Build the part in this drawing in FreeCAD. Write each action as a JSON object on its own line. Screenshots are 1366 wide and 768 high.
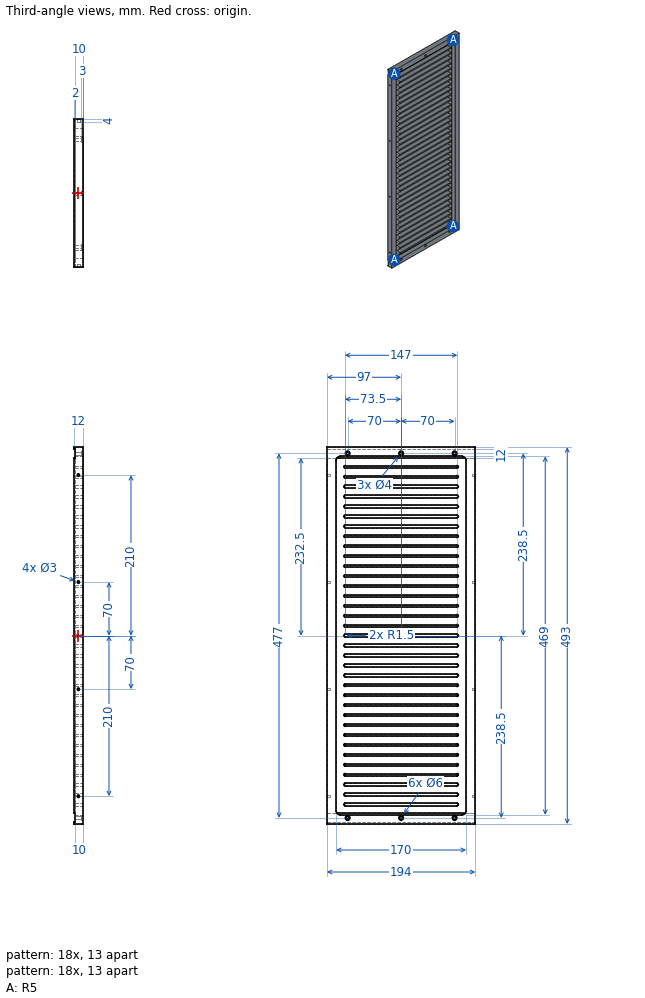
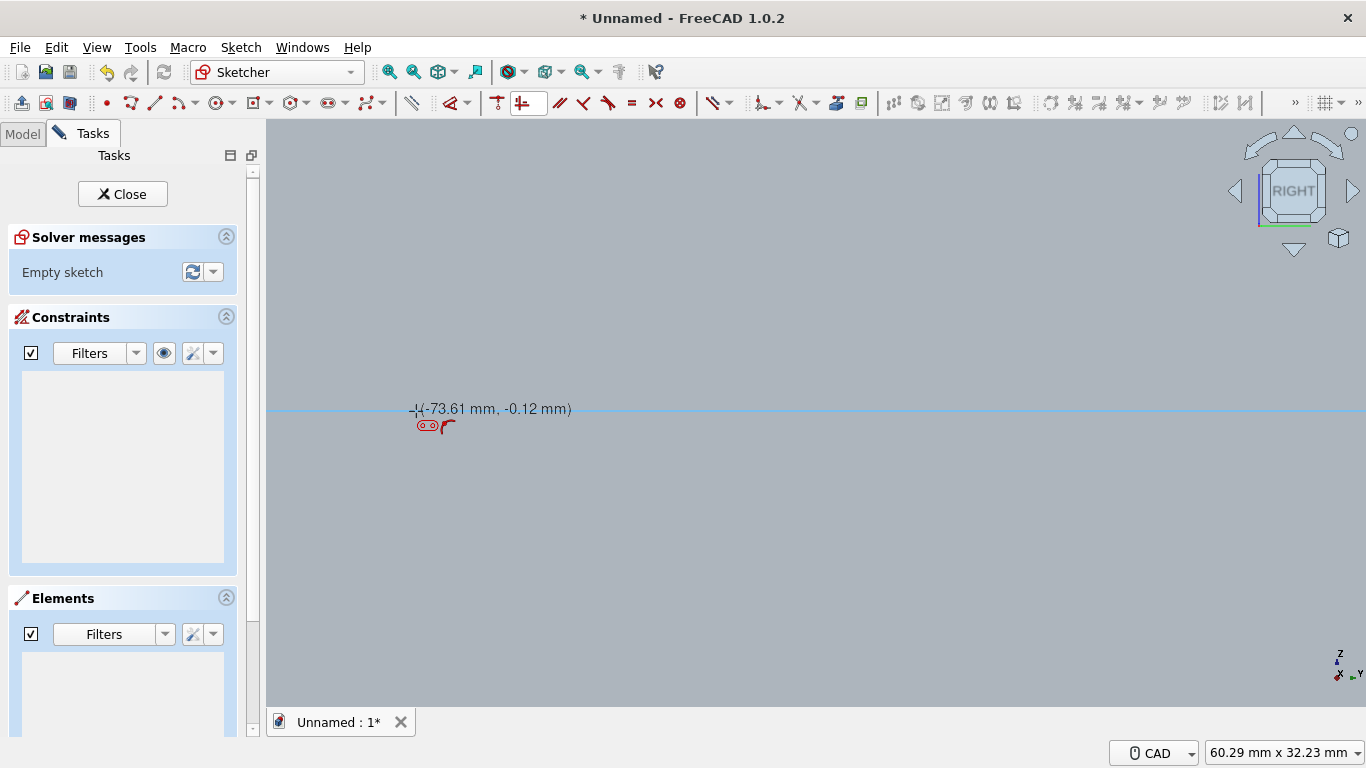
{"action": "scroll", "coordinate": [417, 414], "scroll_direction": "down", "scroll_amount": 7}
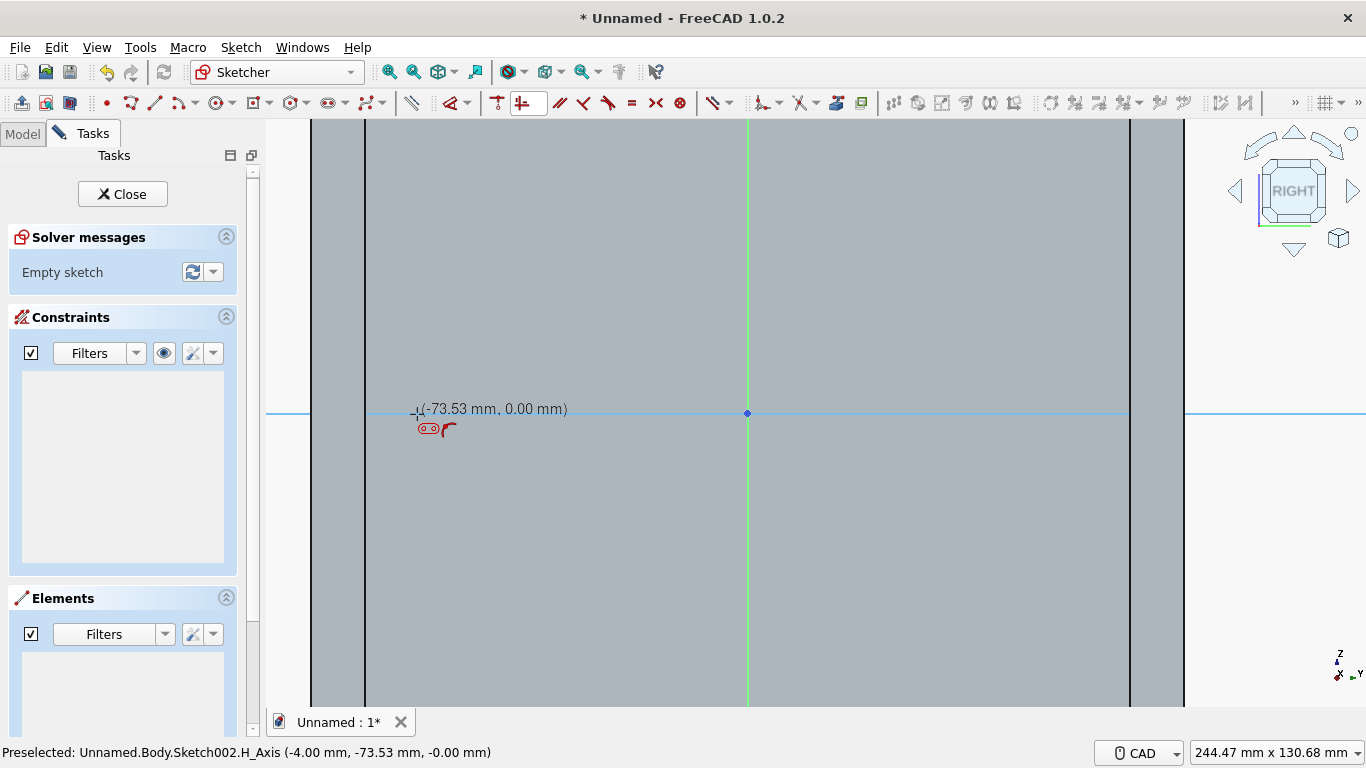
{"action": "left_click", "coordinate": [417, 414]}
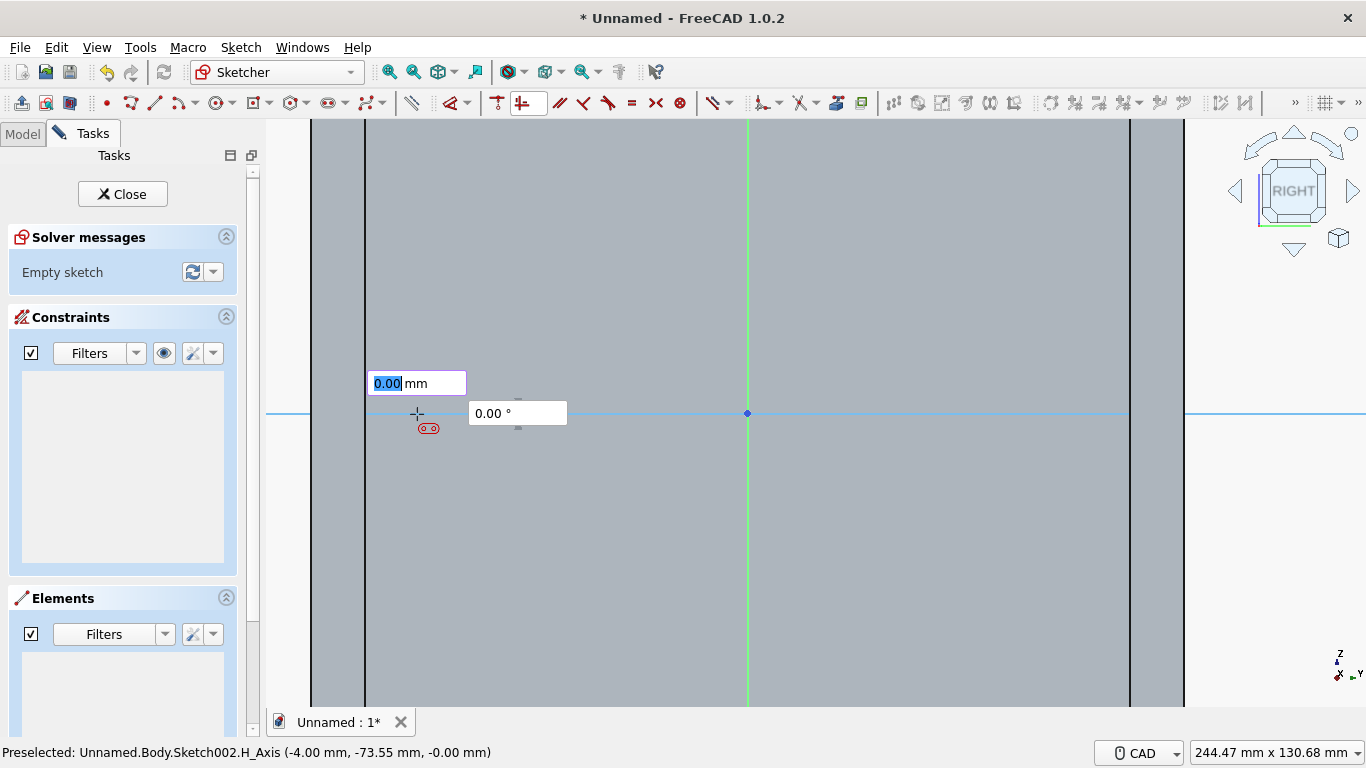
{"action": "left_click", "coordinate": [1079, 405]}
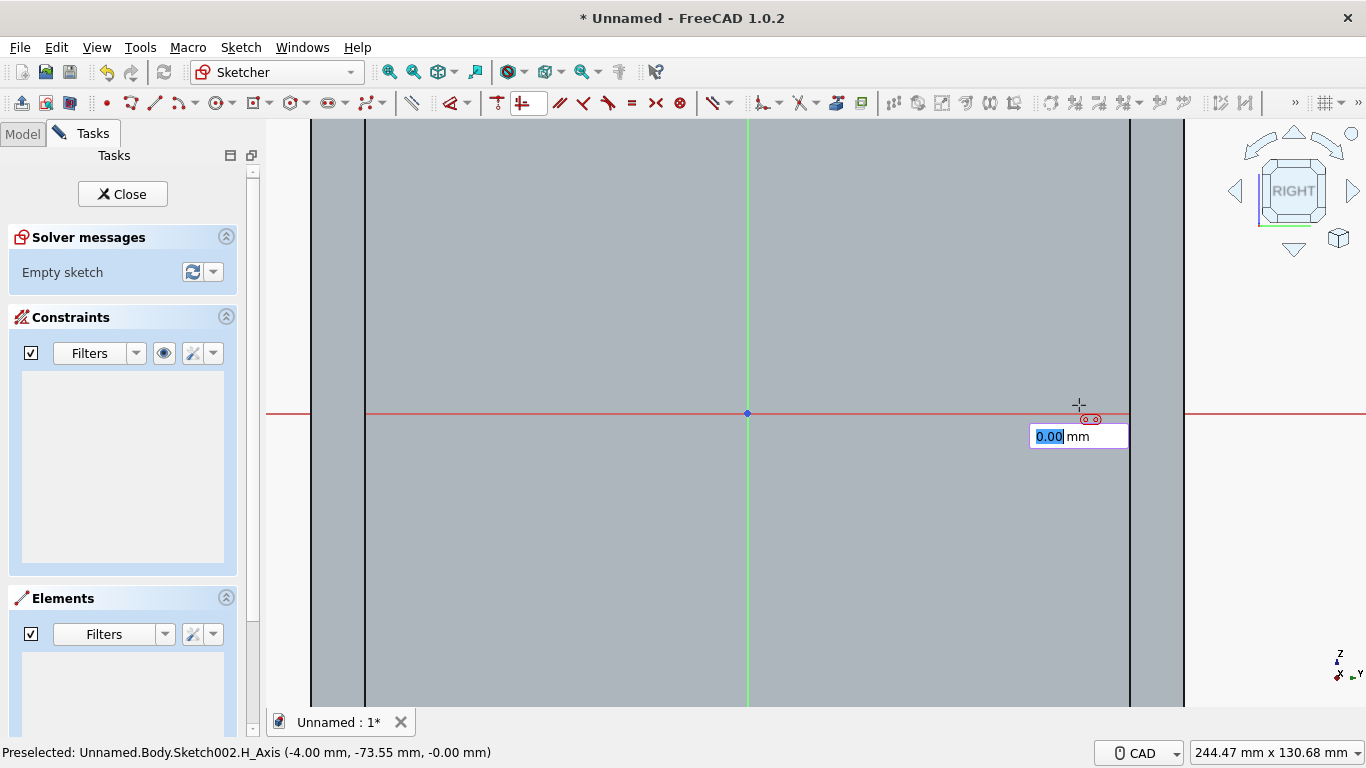
{"action": "scroll", "coordinate": [847, 407], "scroll_direction": "up", "scroll_amount": 5}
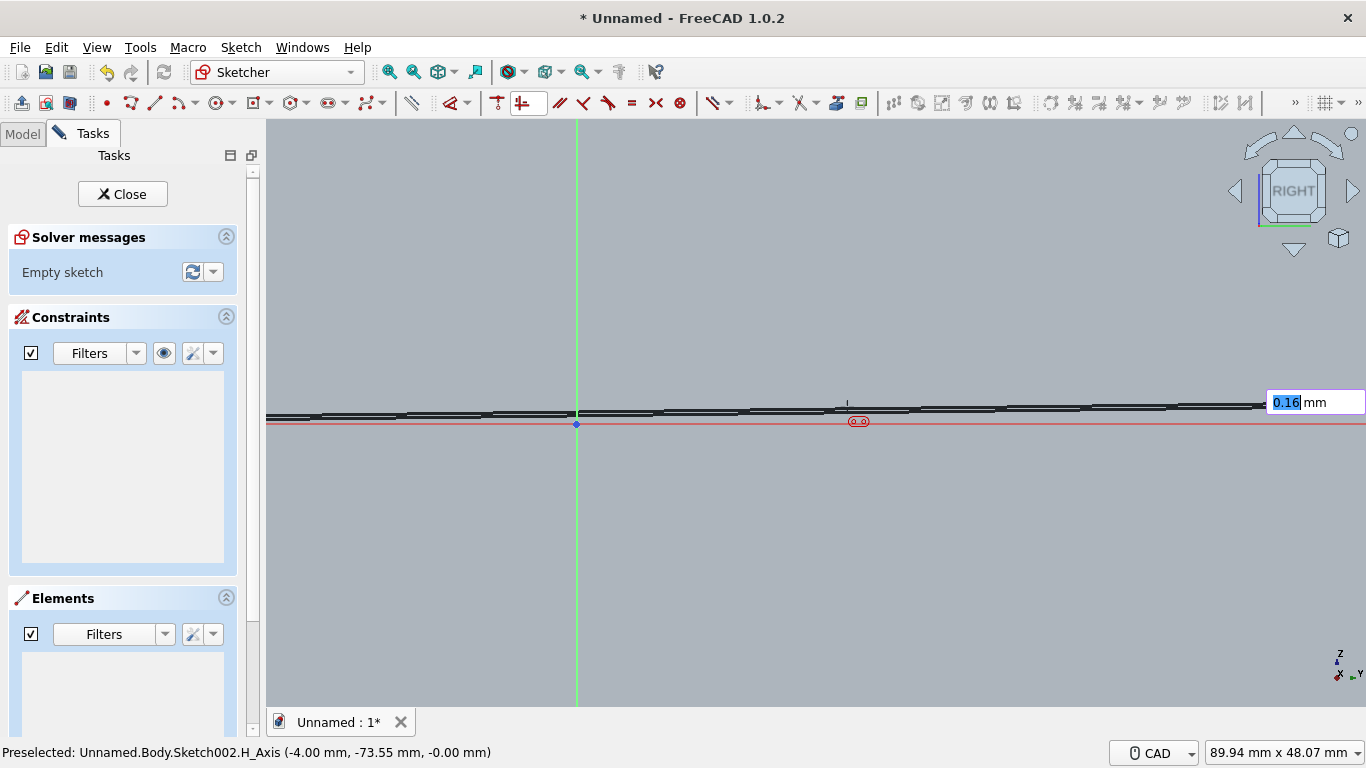
{"action": "left_click", "coordinate": [847, 406]}
{"action": "key", "text": "Escape"}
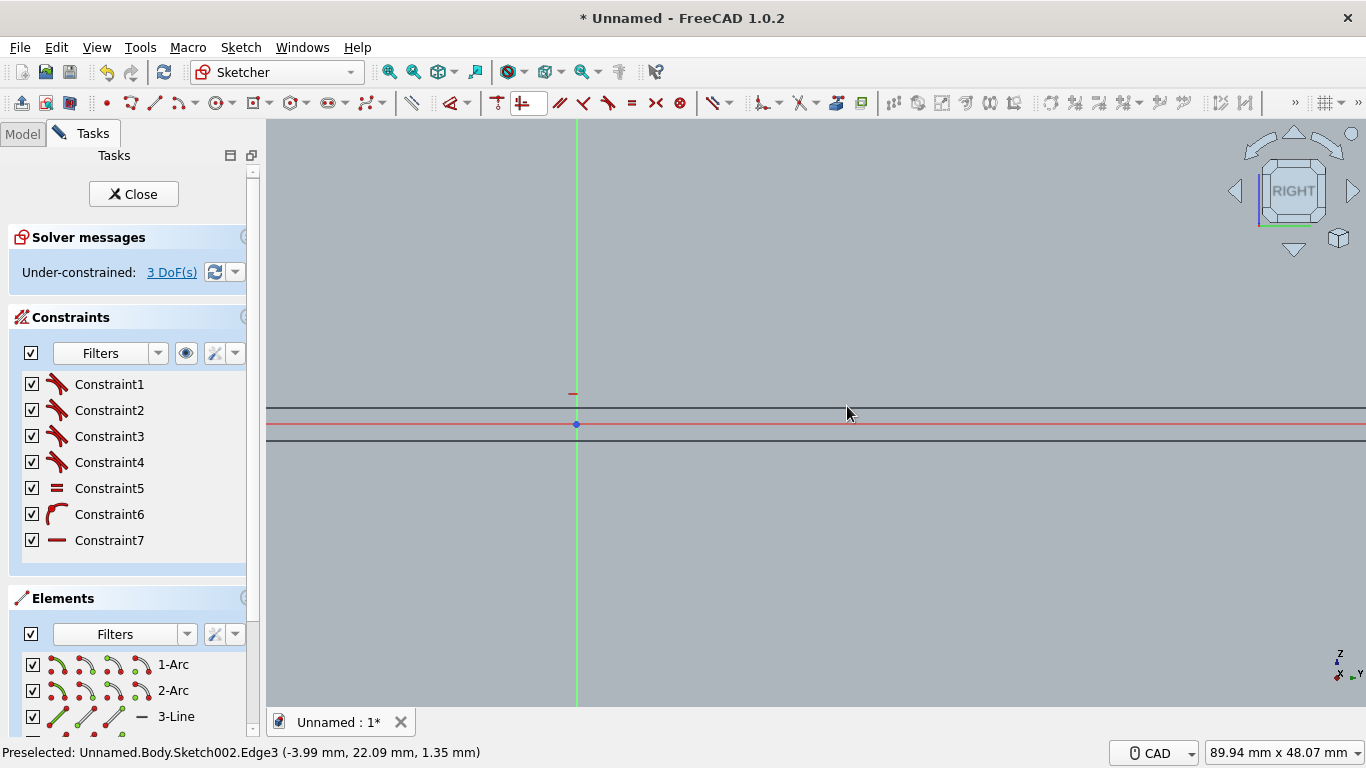
{"action": "scroll", "coordinate": [847, 406], "scroll_direction": "down", "scroll_amount": 5}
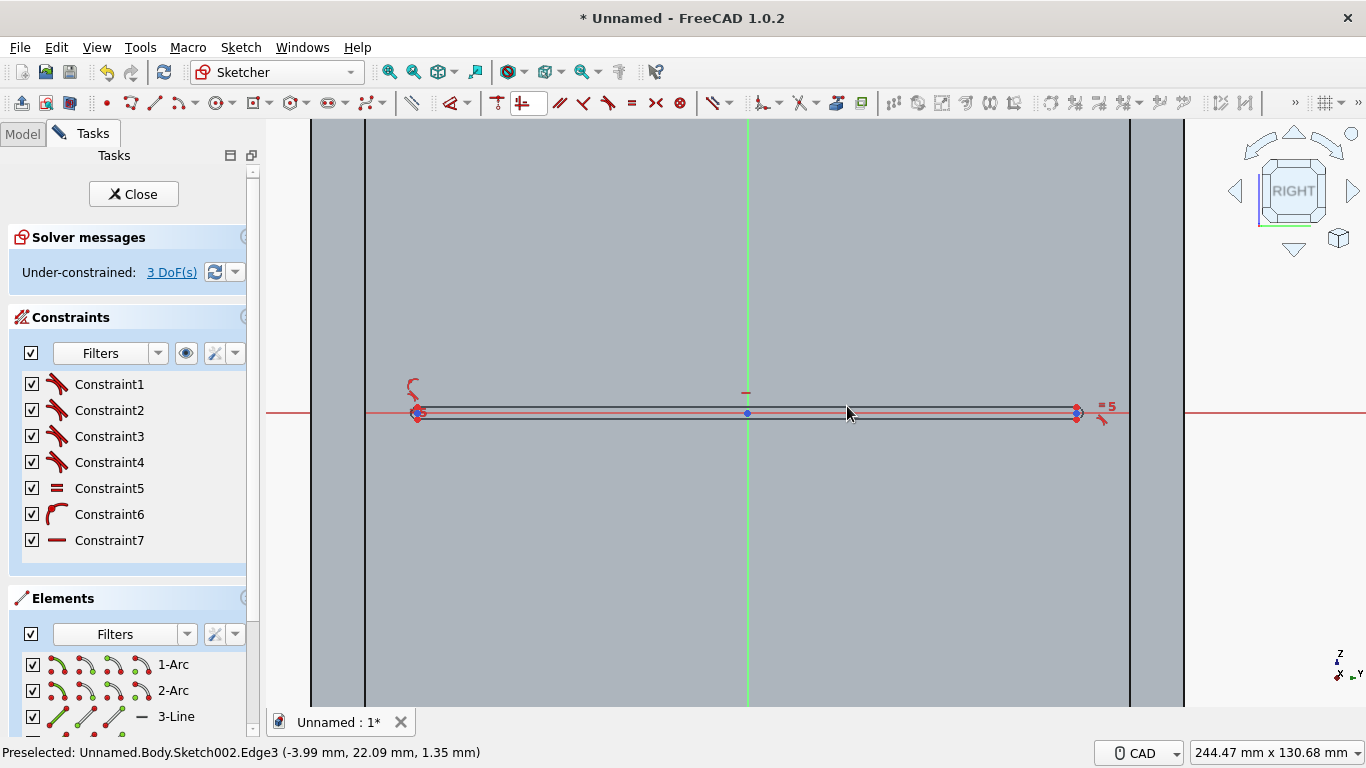
{"action": "scroll", "coordinate": [412, 410], "scroll_direction": "up", "scroll_amount": 9}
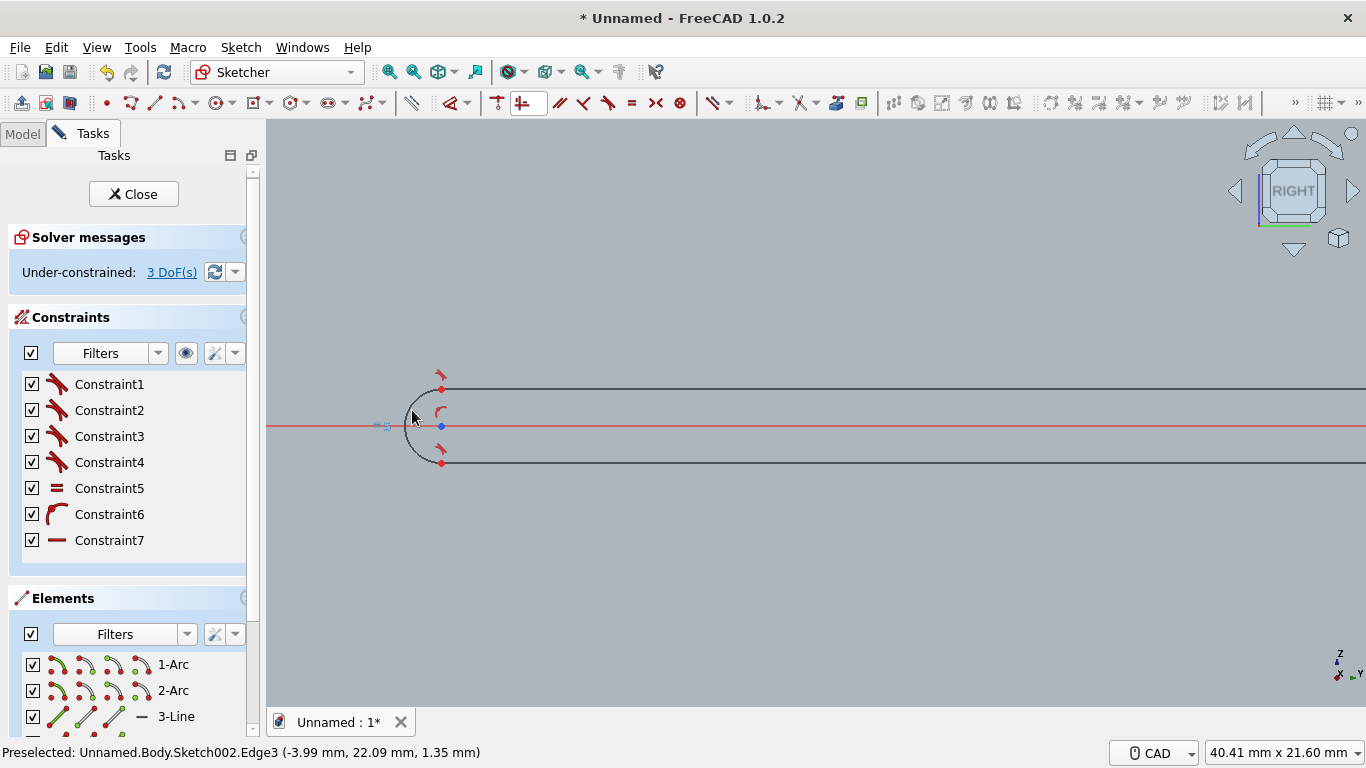
{"action": "left_click", "coordinate": [412, 405]}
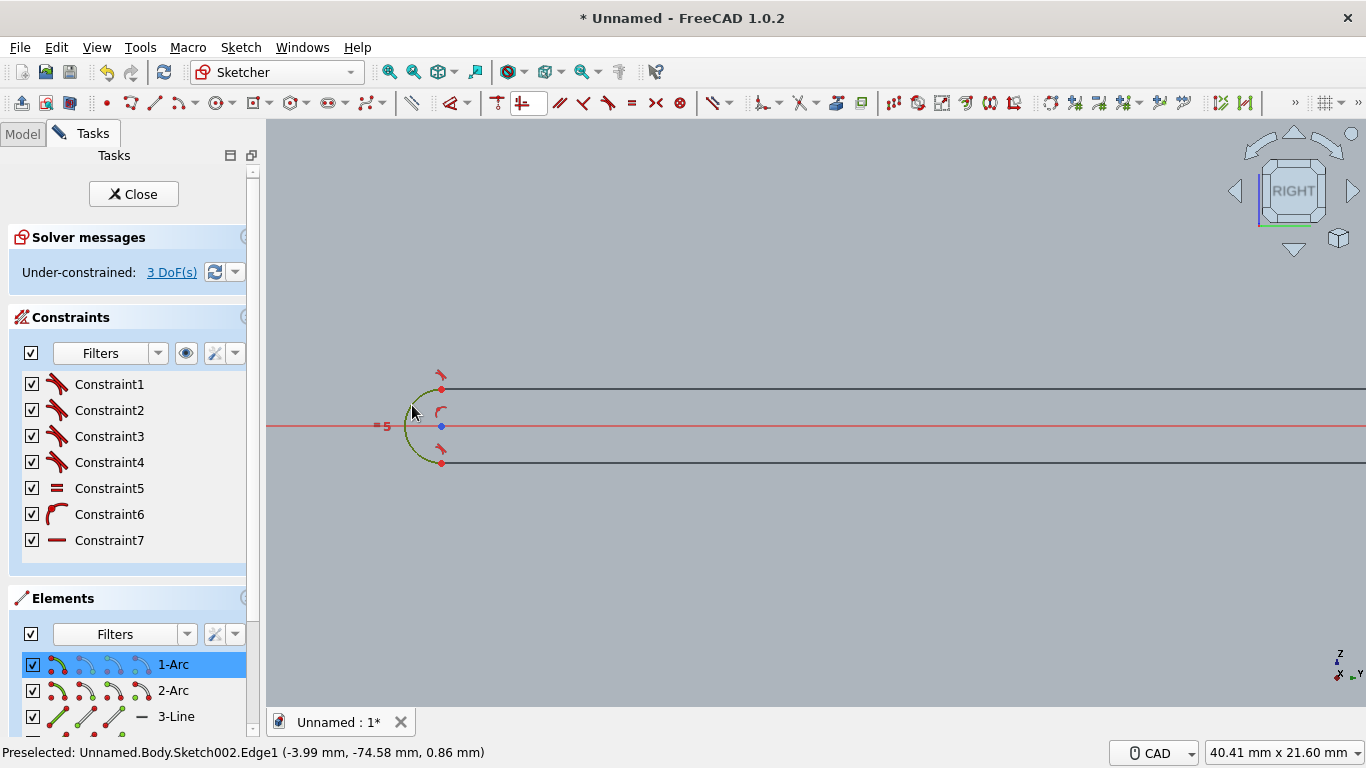
{"action": "key", "text": "k r"}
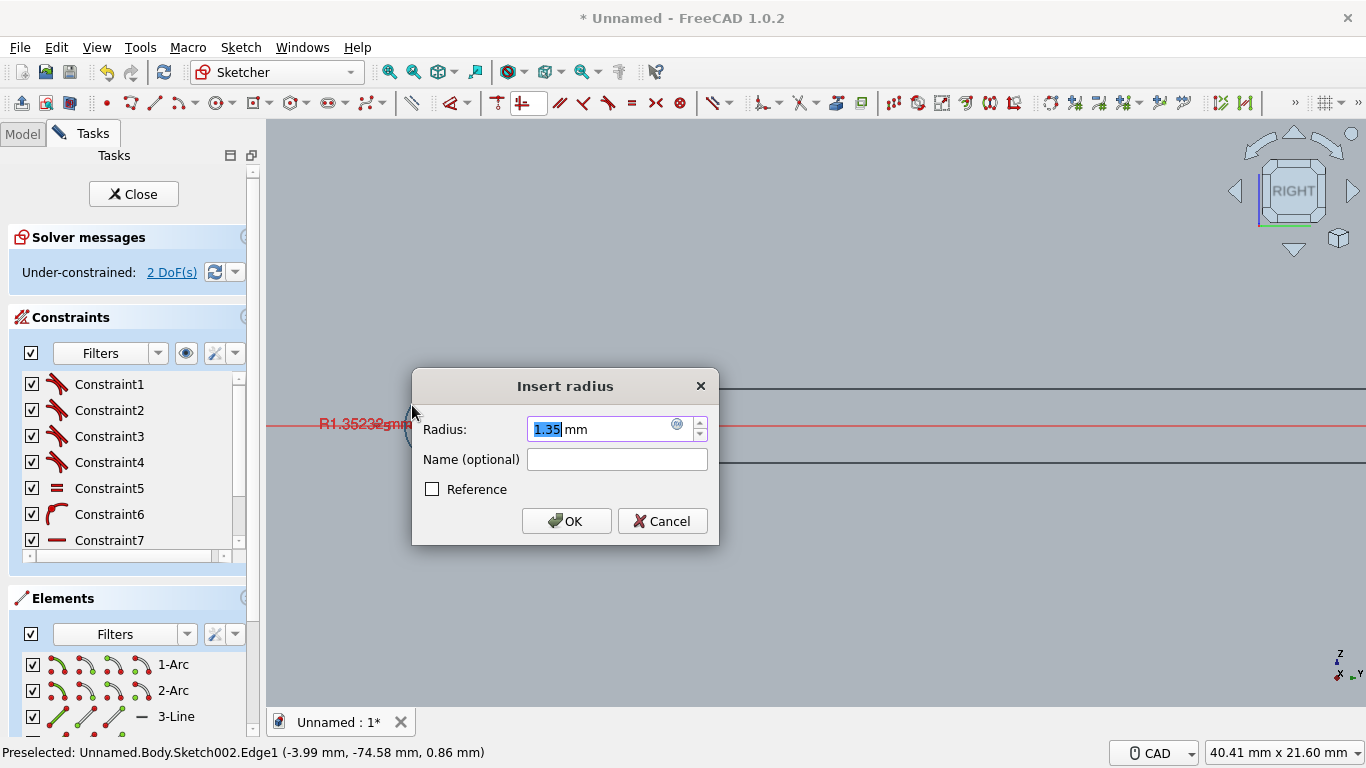
{"action": "type", "text": "1.5"}
{"action": "key", "text": "Return"}